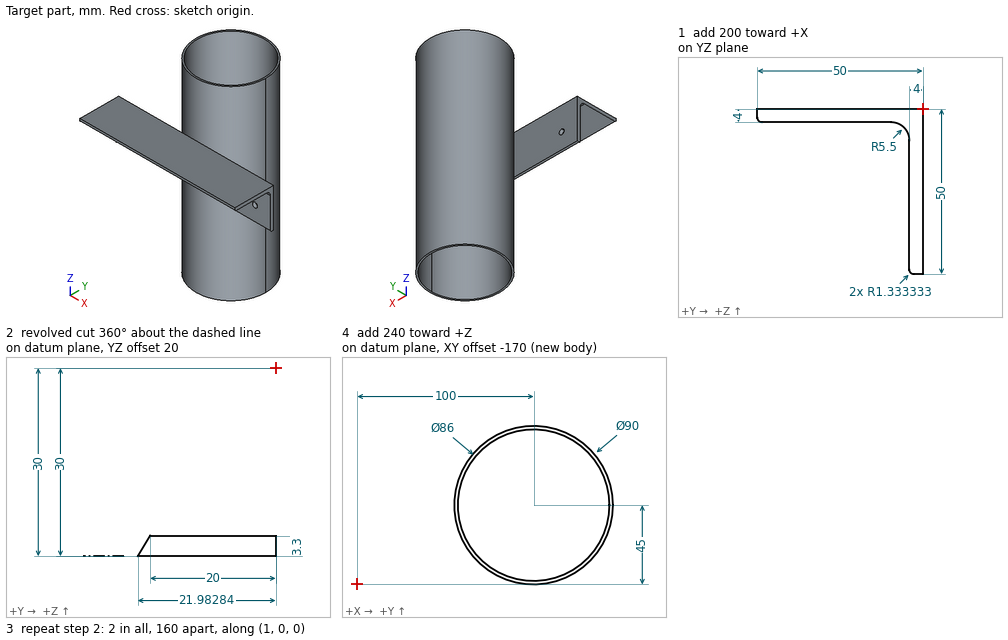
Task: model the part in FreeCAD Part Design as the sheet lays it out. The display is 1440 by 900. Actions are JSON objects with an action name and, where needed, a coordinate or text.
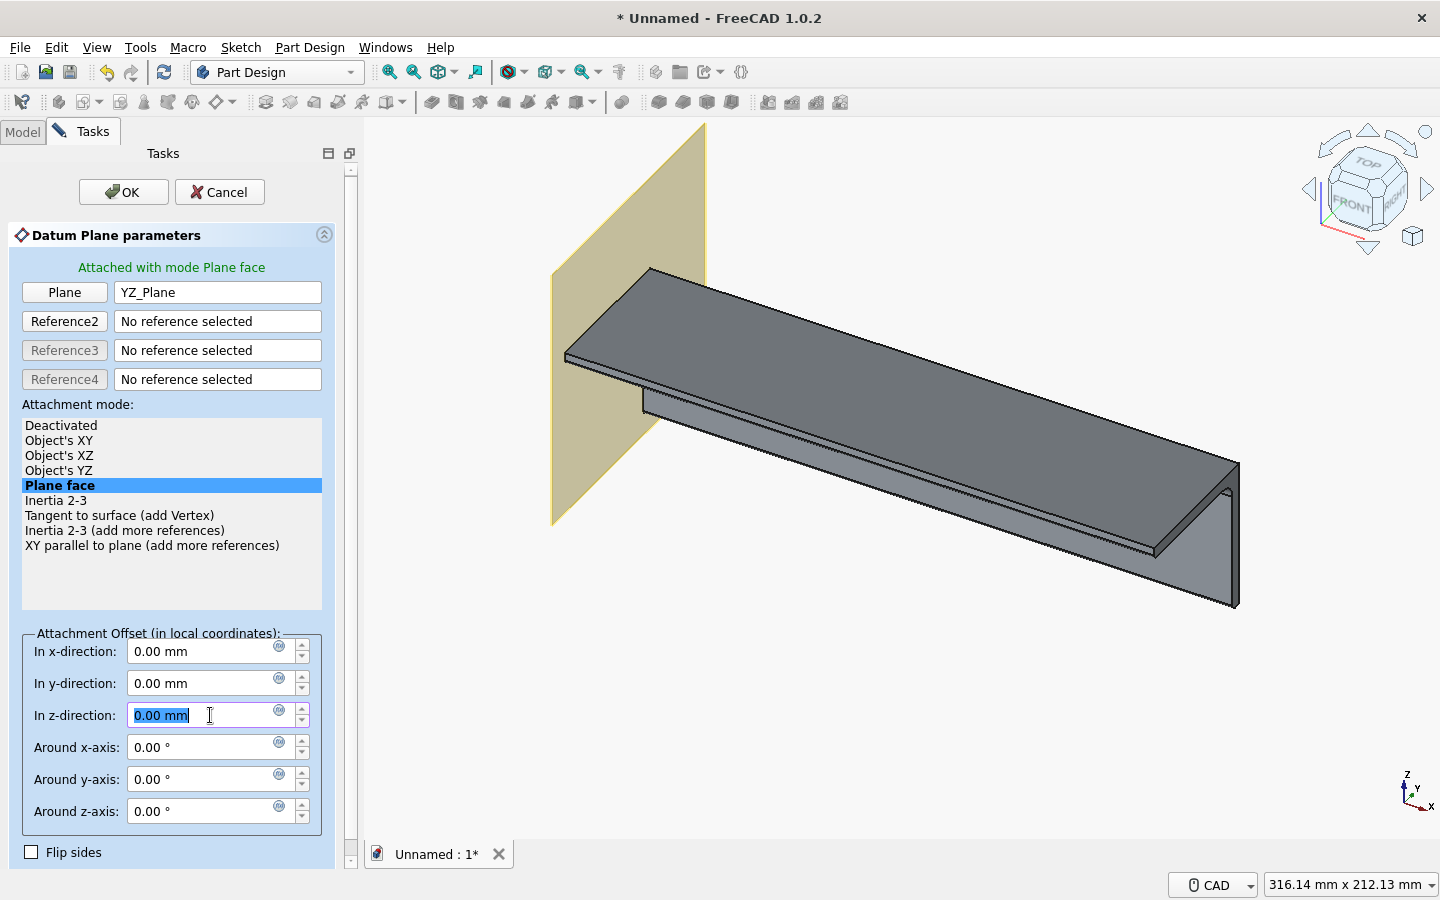
{"action": "type", "text": "20"}
{"action": "key", "text": "Tab"}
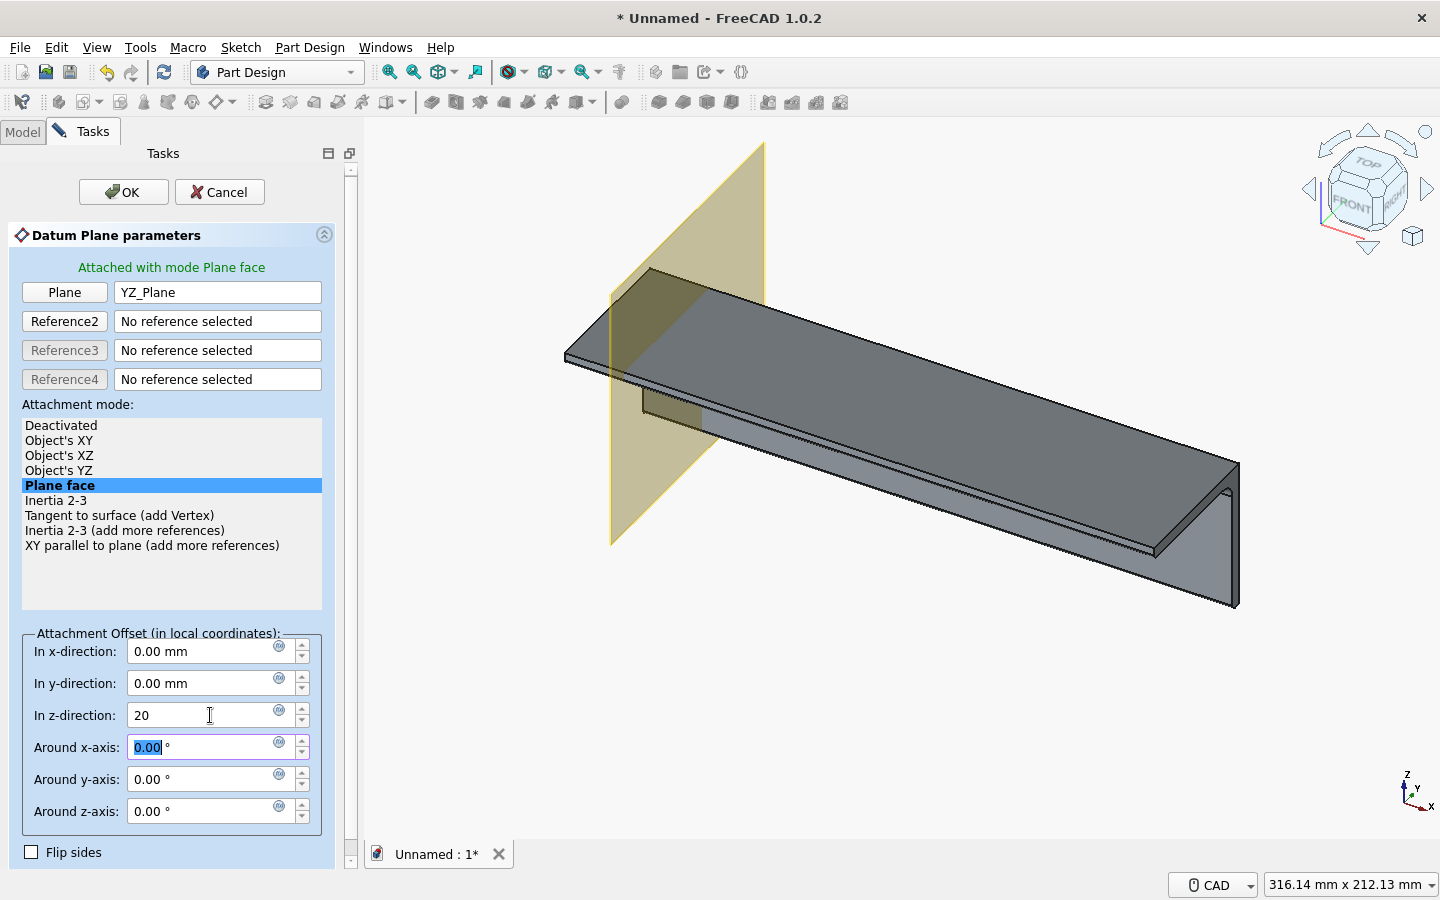
{"action": "left_click", "coordinate": [124, 192]}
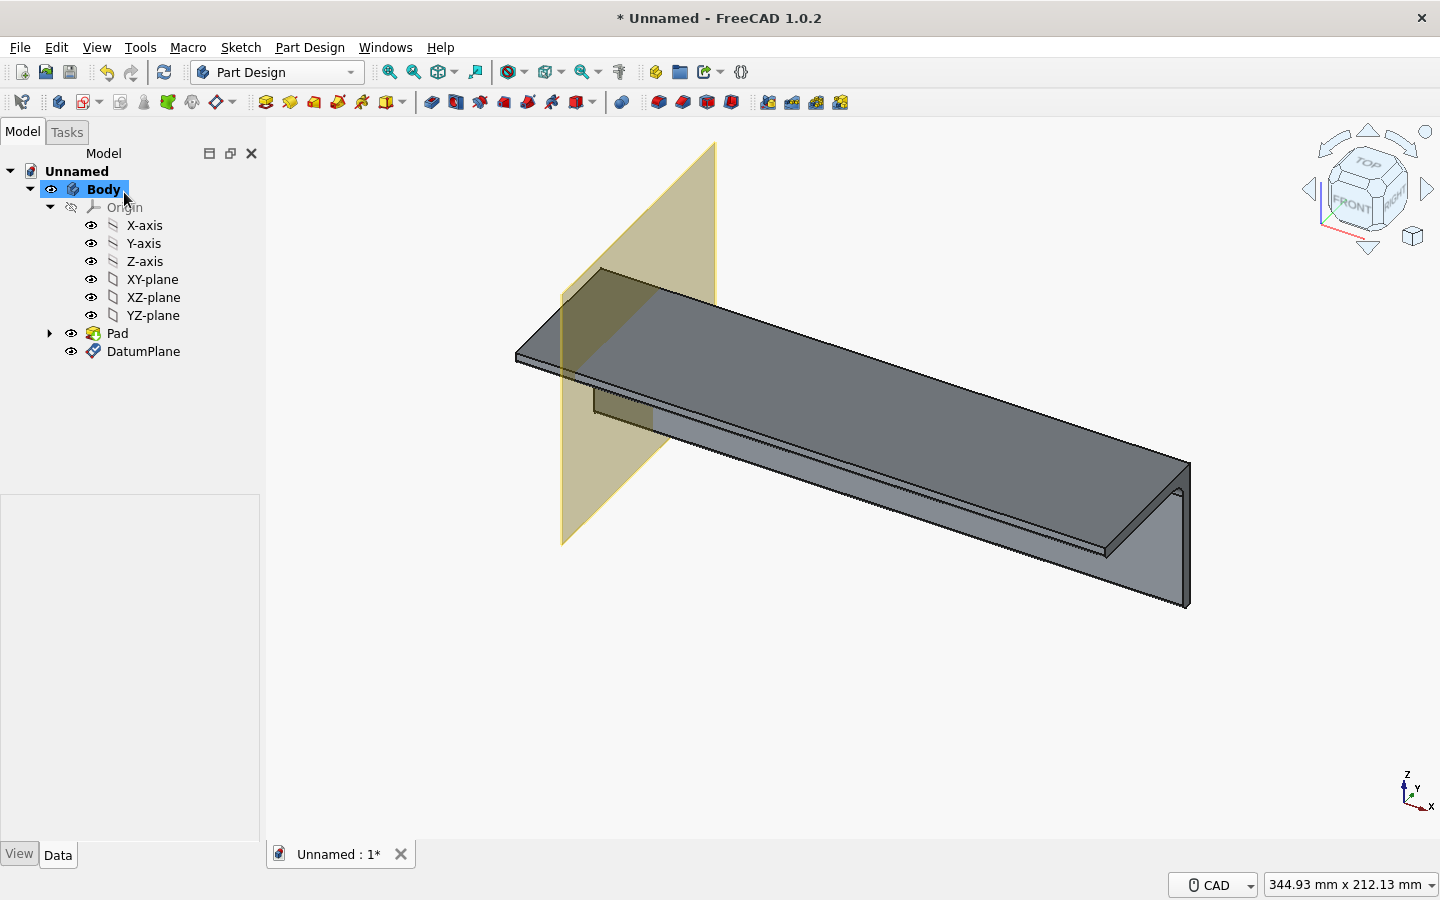
{"action": "left_click", "coordinate": [116, 351]}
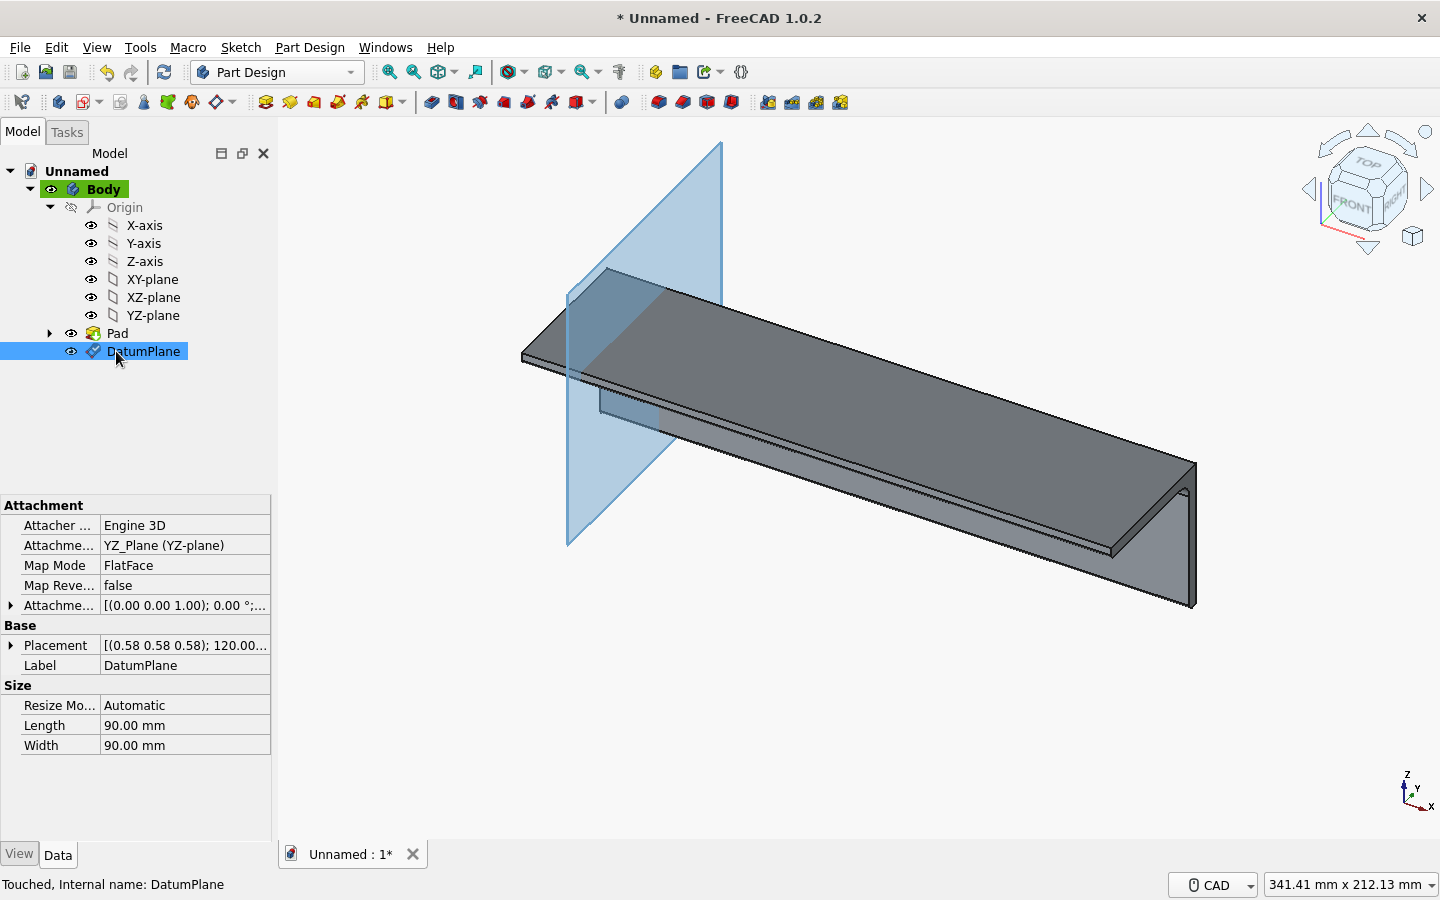
{"action": "left_click", "coordinate": [84, 102]}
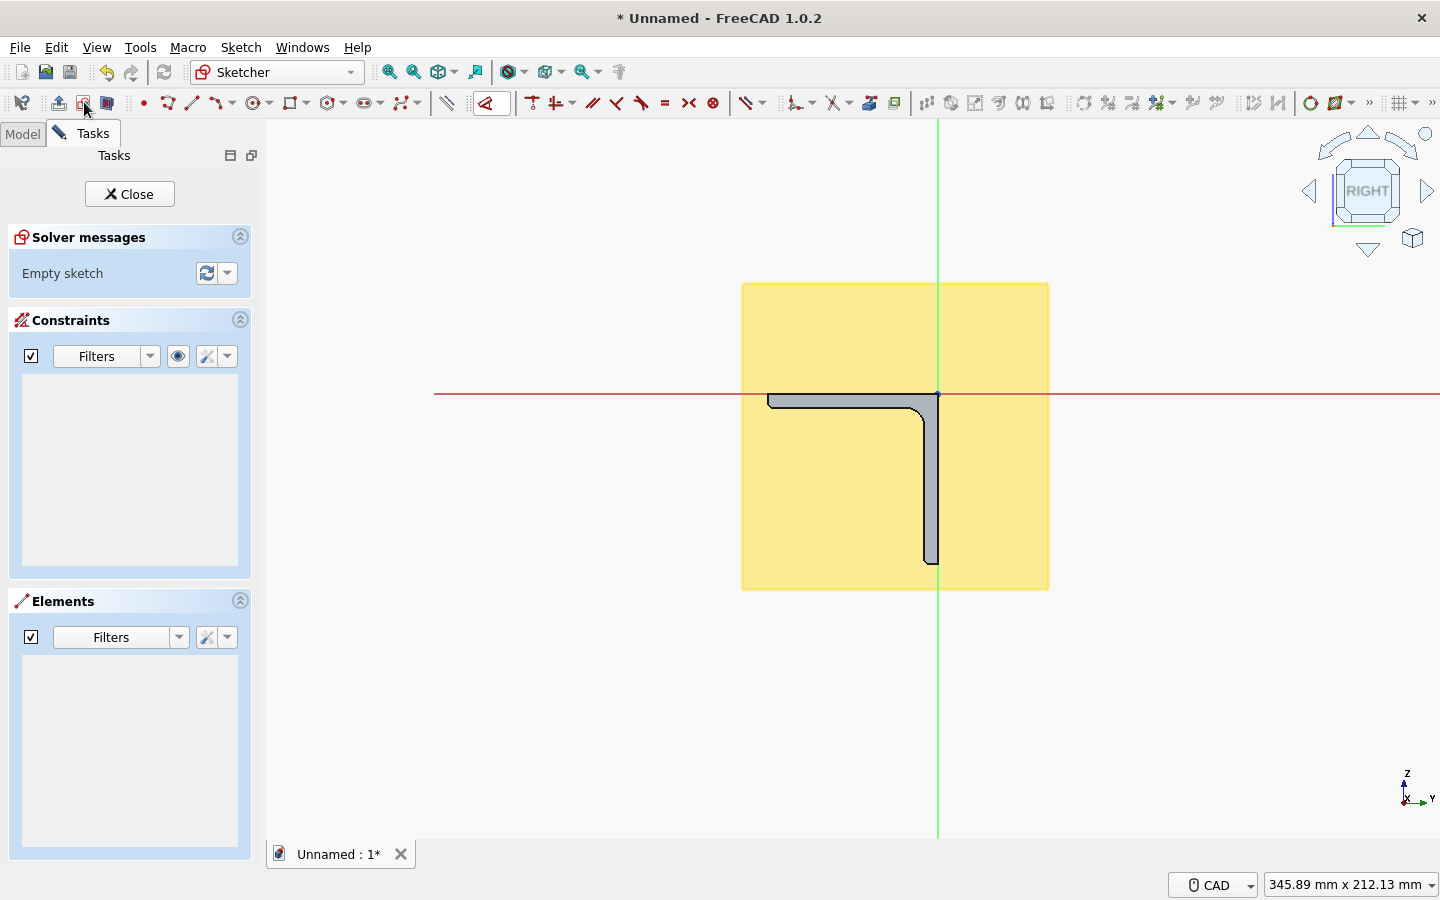
{"action": "left_click", "coordinate": [108, 104]}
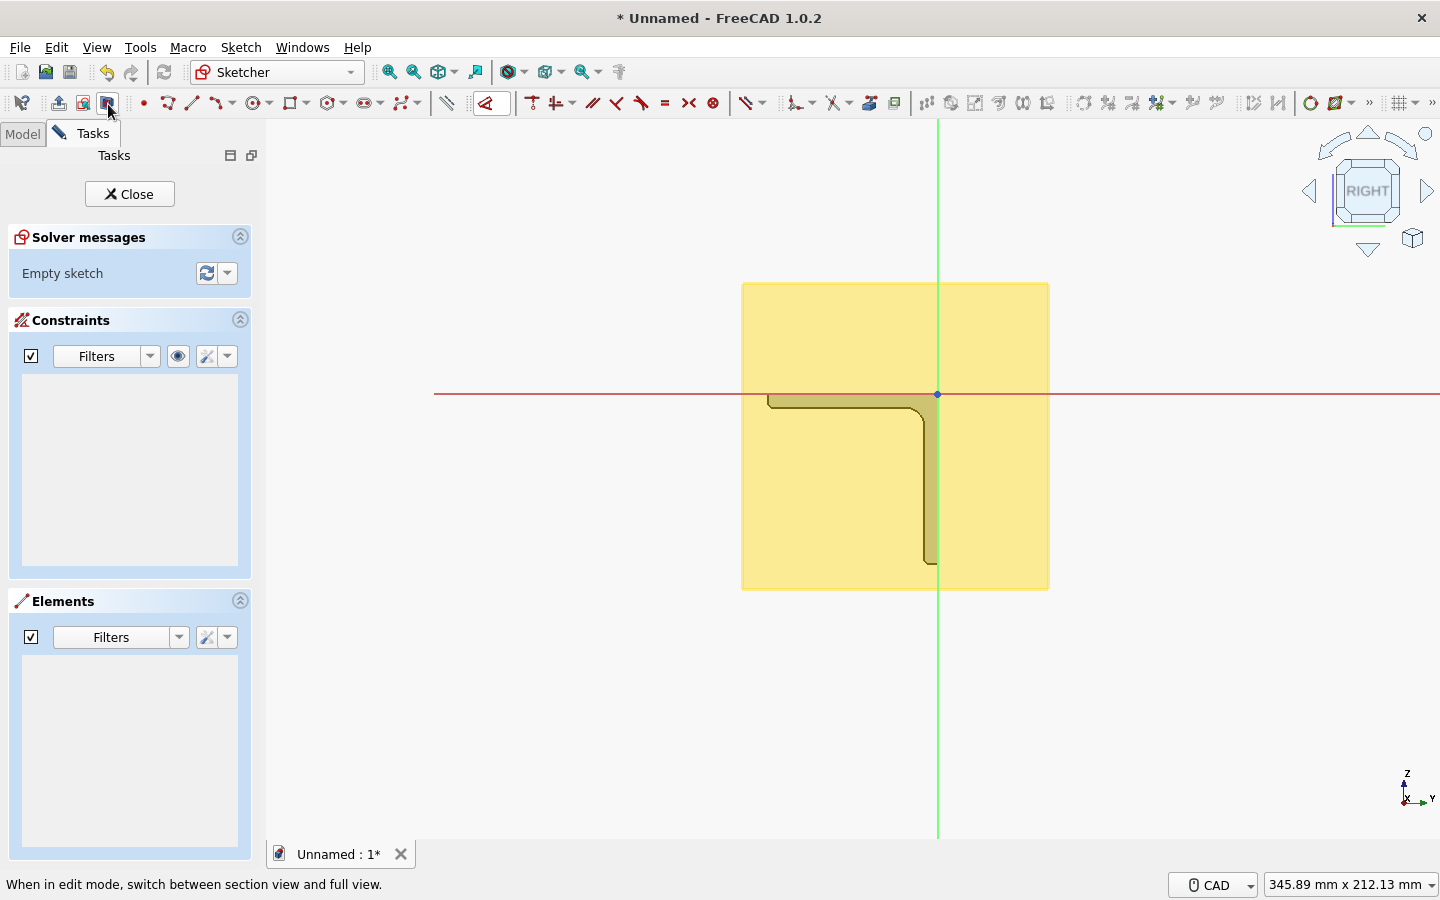
{"action": "scroll", "coordinate": [911, 436], "scroll_direction": "up", "scroll_amount": 8}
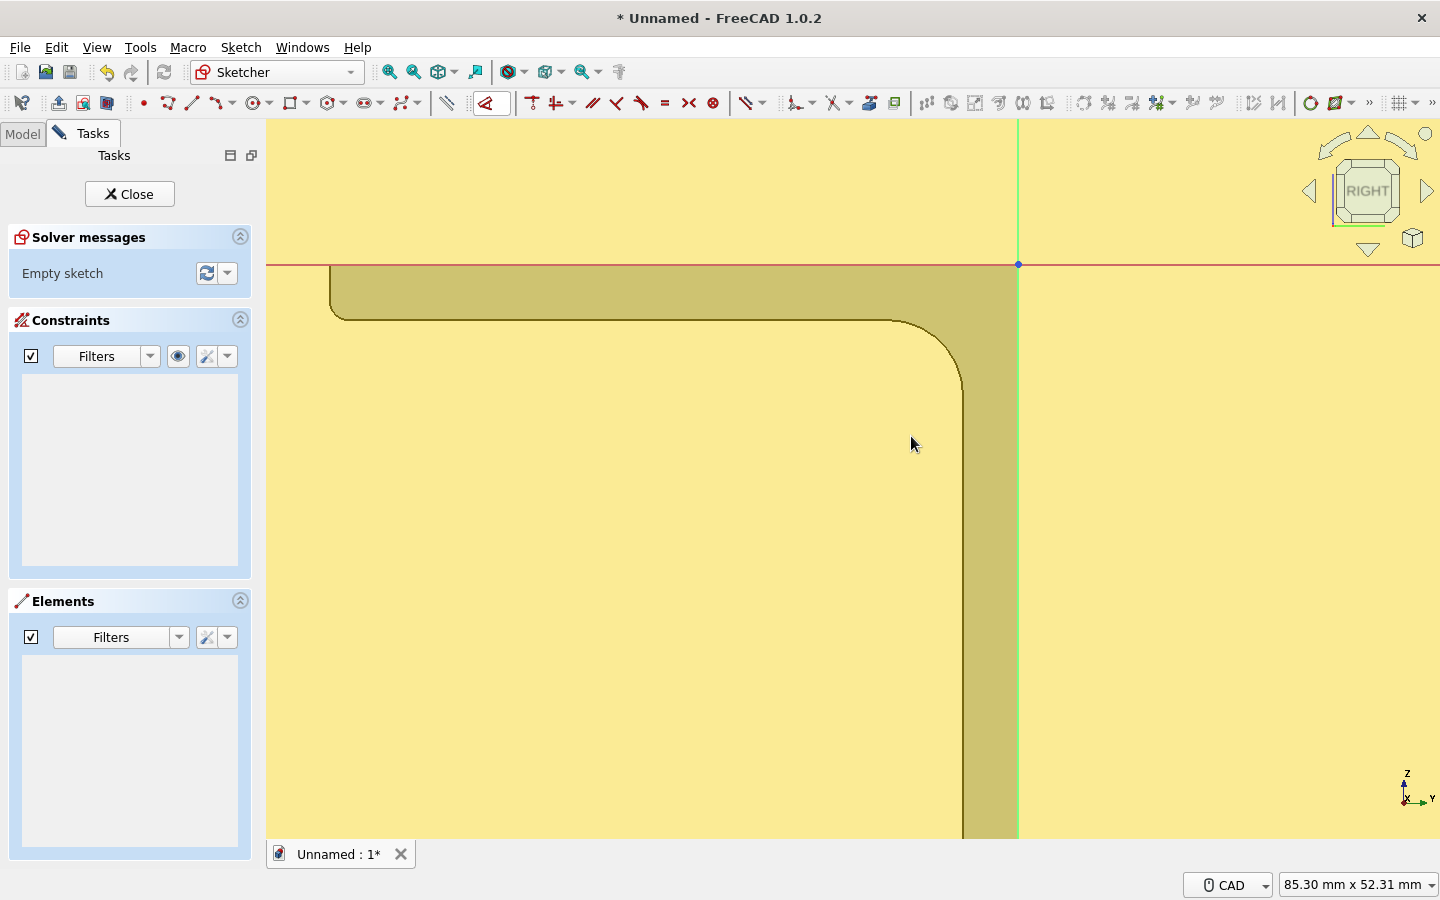
{"action": "left_click", "coordinate": [168, 104]}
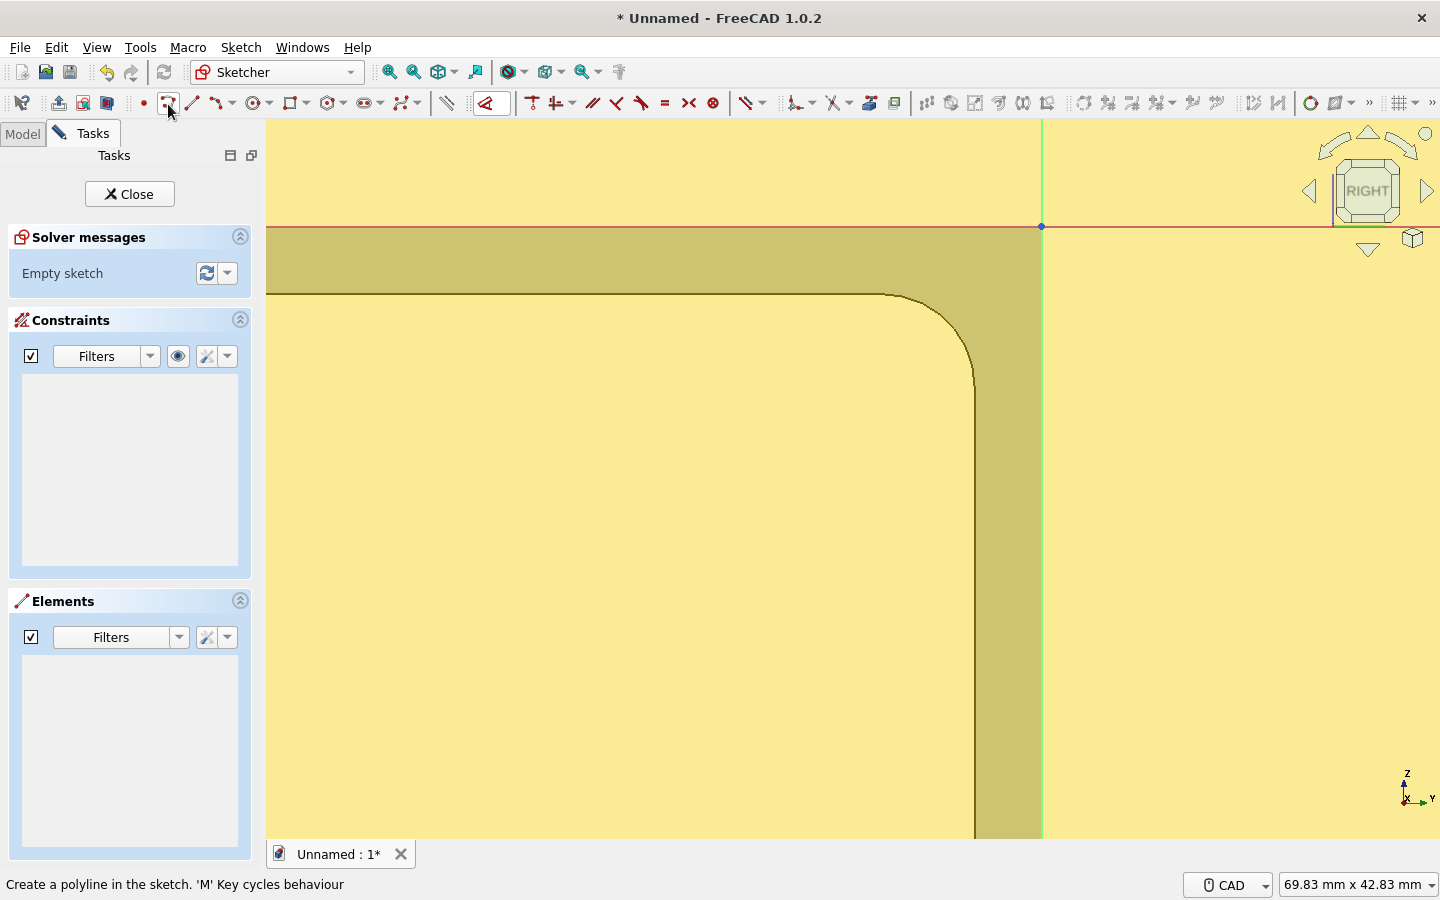
{"action": "left_click", "coordinate": [1042, 676]}
{"action": "left_click", "coordinate": [706, 676]}
{"action": "left_click", "coordinate": [672, 731]}
{"action": "left_click", "coordinate": [1033, 731]}
{"action": "left_click", "coordinate": [1042, 677]}